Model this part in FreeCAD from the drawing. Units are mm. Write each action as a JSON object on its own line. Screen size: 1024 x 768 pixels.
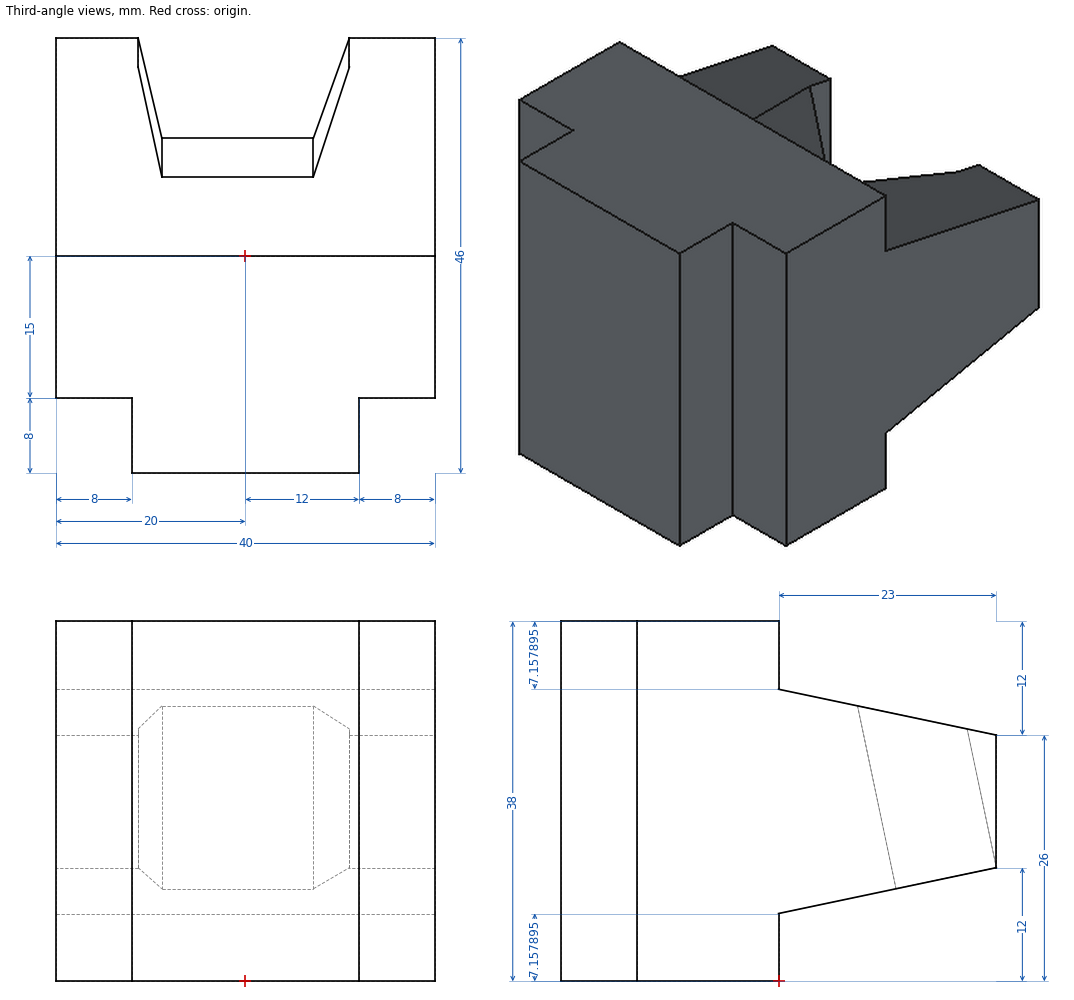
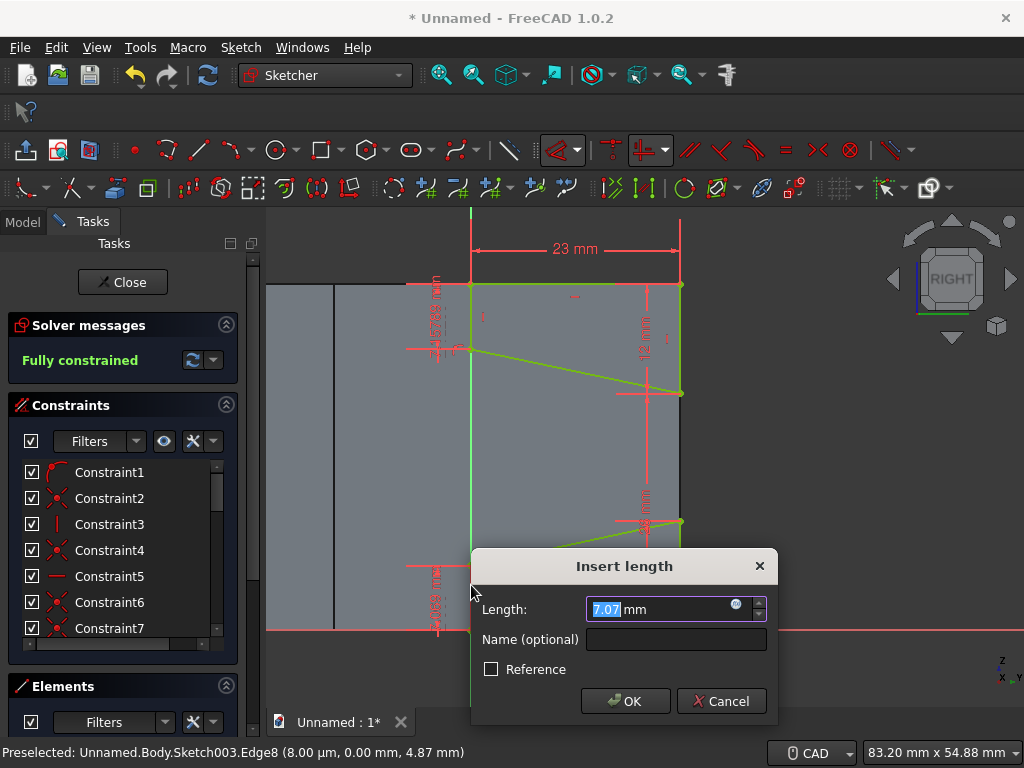
{"action": "type", "text": "7.157895"}
{"action": "key", "text": "Return"}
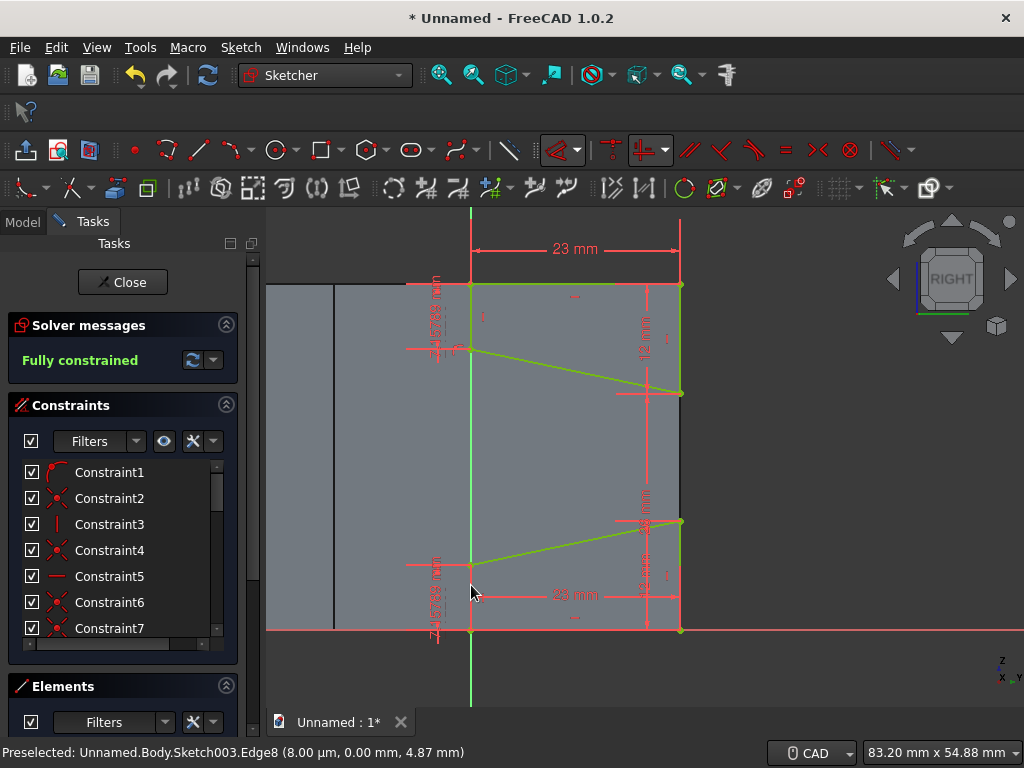
{"action": "left_click", "coordinate": [123, 282]}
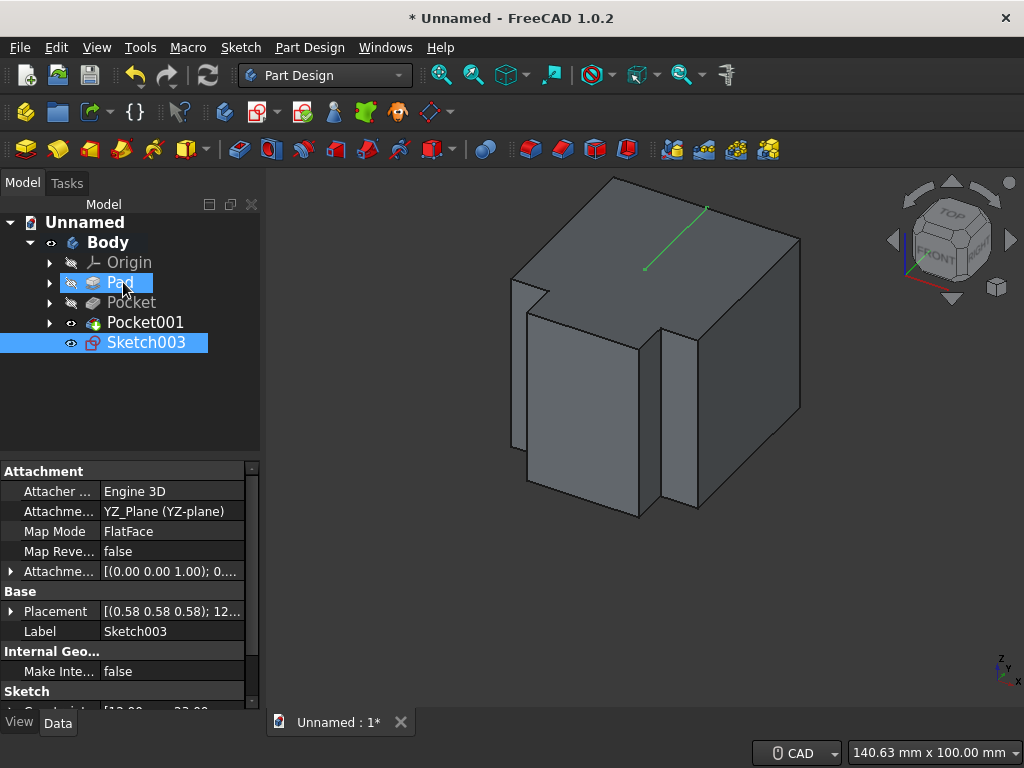
{"action": "left_click", "coordinate": [240, 150]}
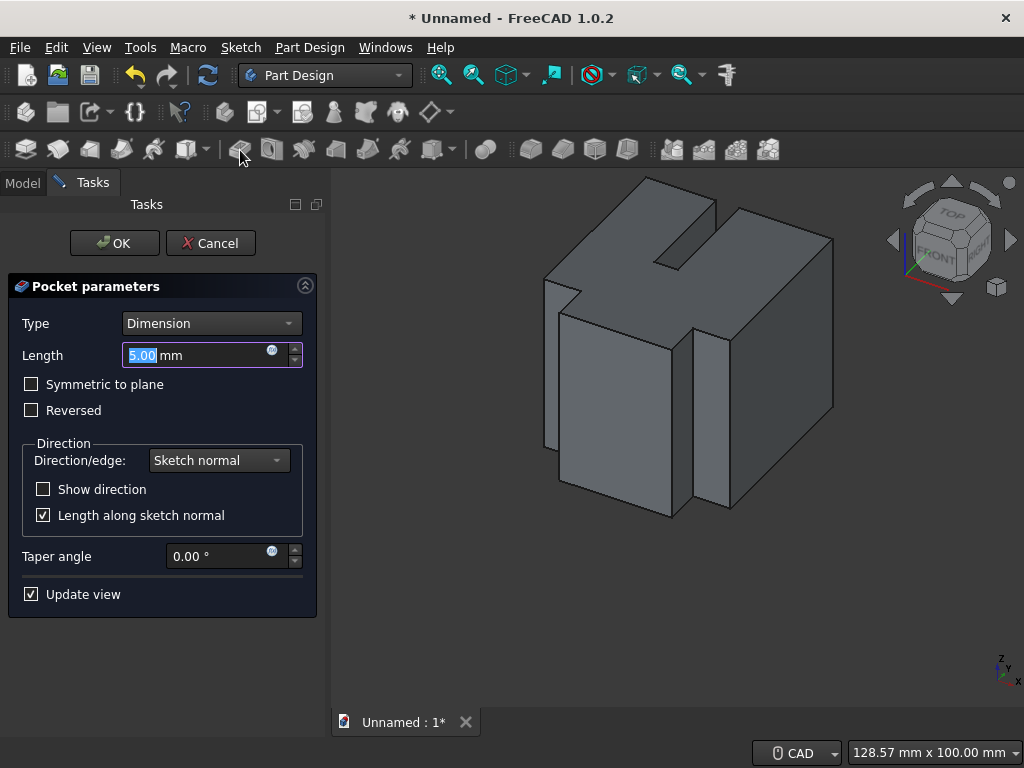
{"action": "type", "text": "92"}
{"action": "key", "text": "Tab"}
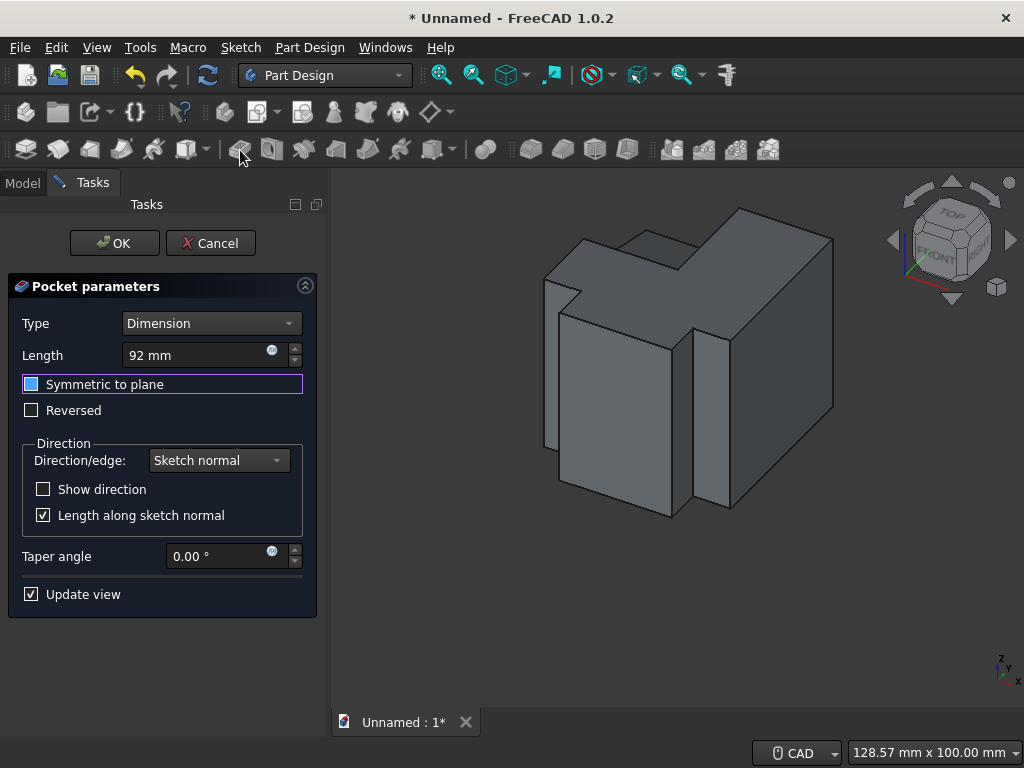
{"action": "left_click", "coordinate": [30, 384]}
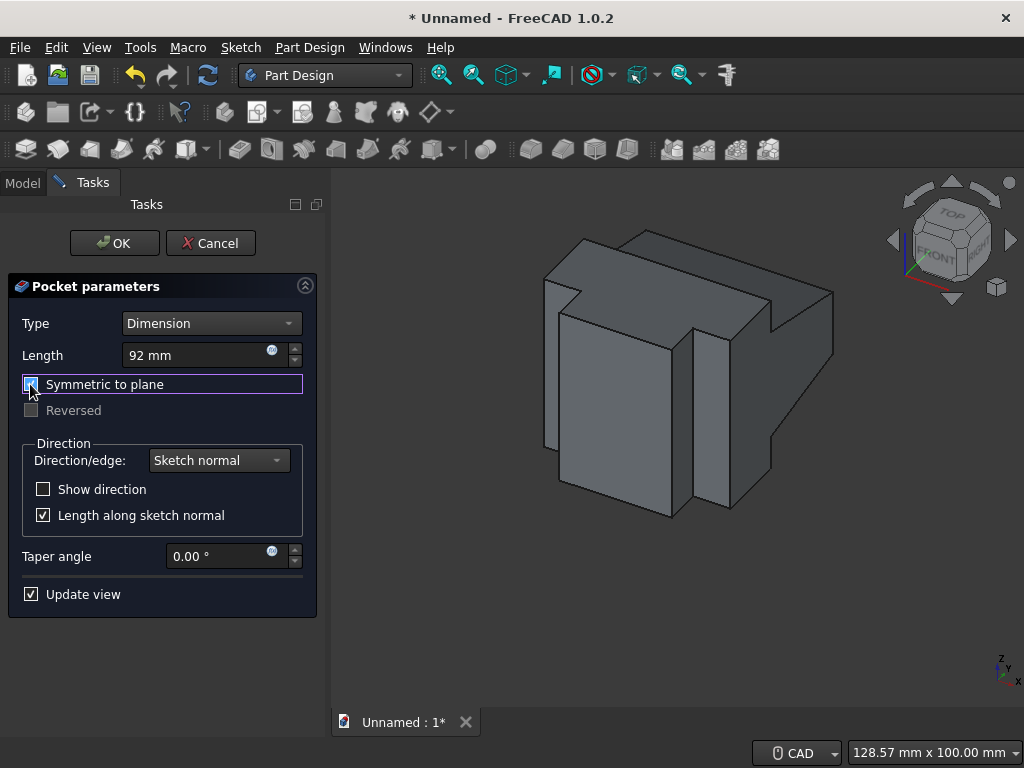
{"action": "left_click", "coordinate": [115, 243]}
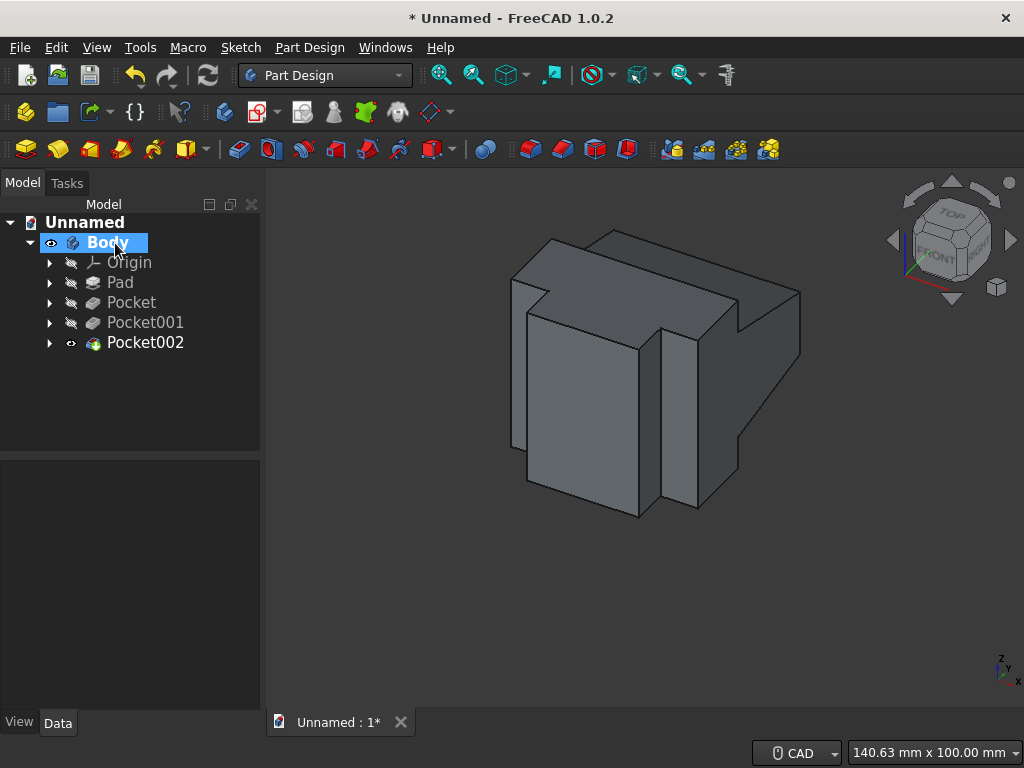
{"action": "key", "text": "5"}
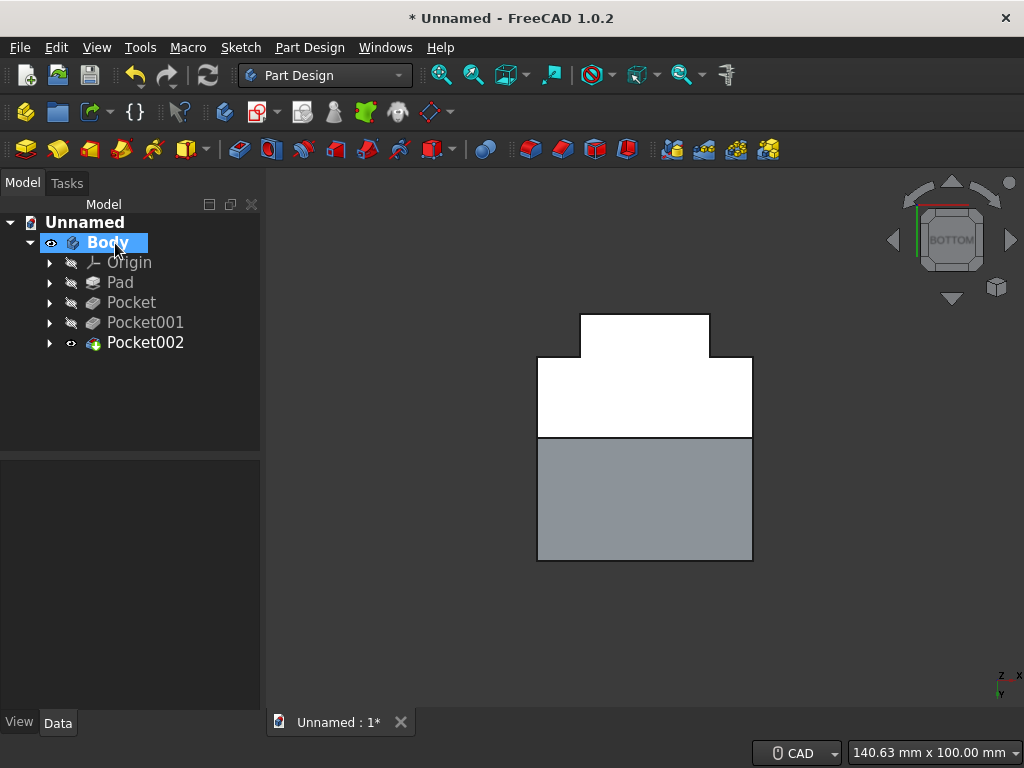
{"action": "left_click", "coordinate": [676, 498]}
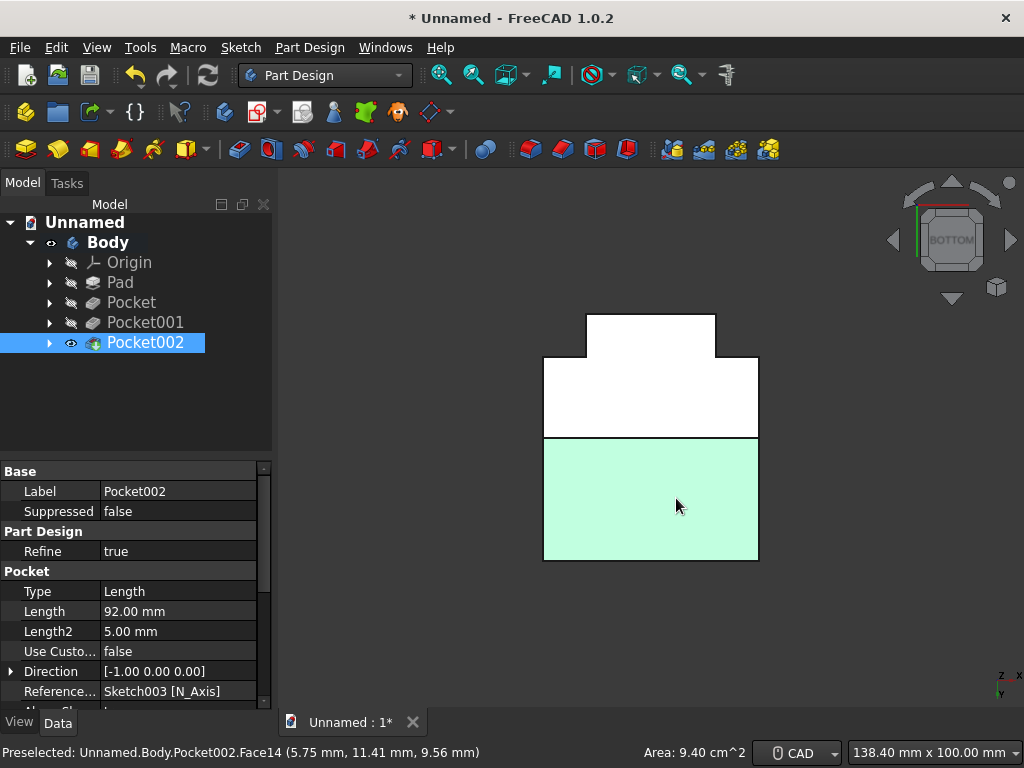
{"action": "left_click", "coordinate": [258, 112]}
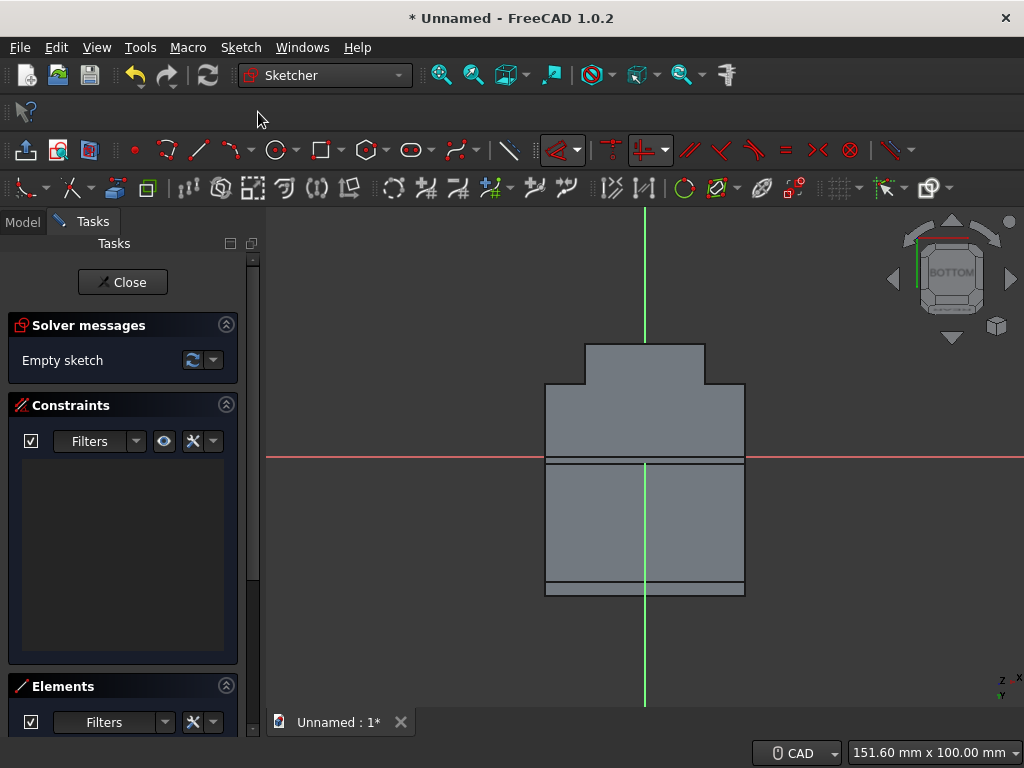
{"action": "scroll", "coordinate": [684, 556], "scroll_direction": "up", "scroll_amount": 5}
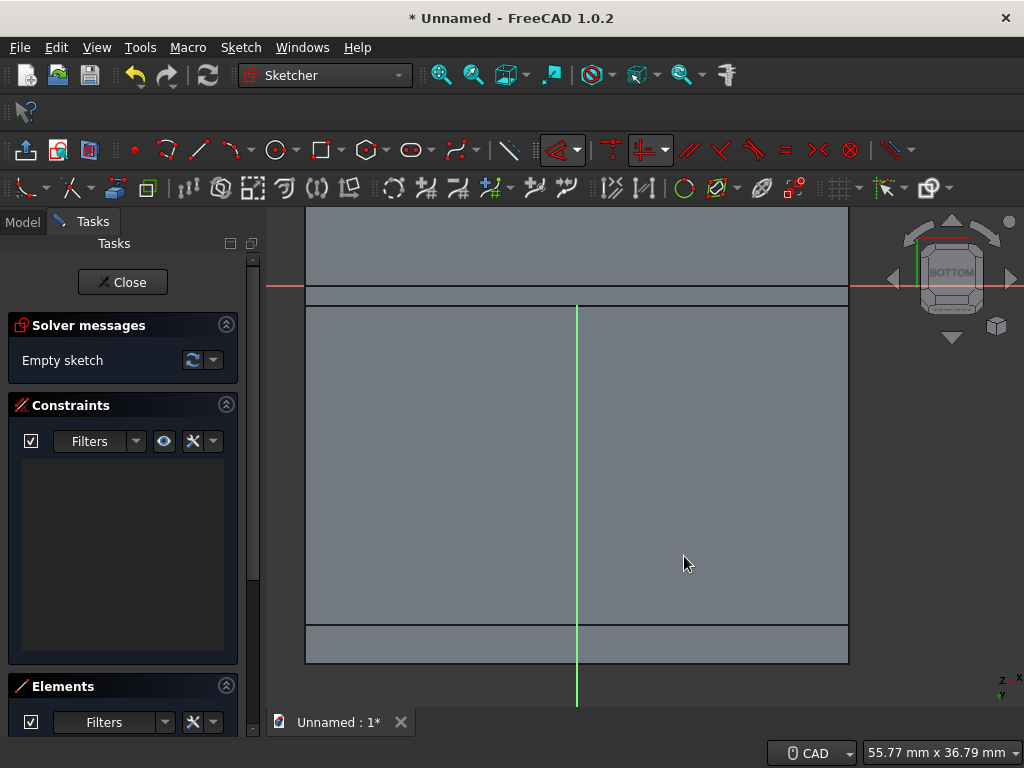
{"action": "left_click", "coordinate": [168, 150]}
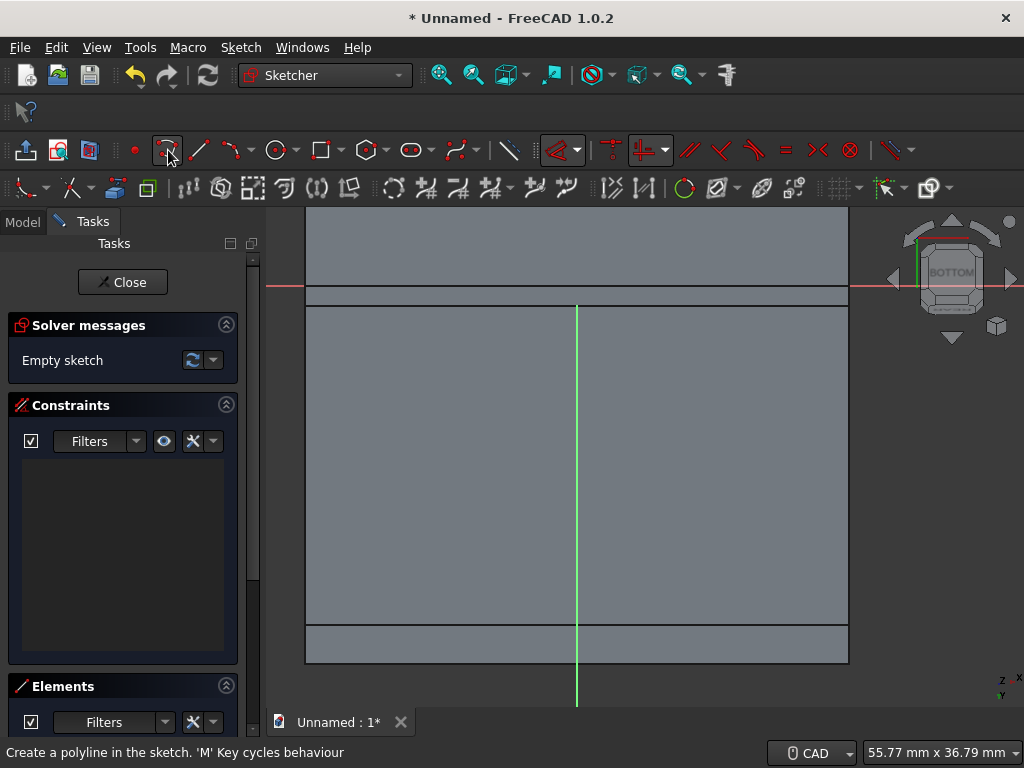
{"action": "left_click", "coordinate": [675, 478]}
{"action": "left_click", "coordinate": [457, 478]}
{"action": "left_click", "coordinate": [423, 625]}
{"action": "left_click", "coordinate": [726, 625]}
{"action": "left_click", "coordinate": [675, 479]}
{"action": "key", "text": "Escape"}
{"action": "key", "text": "Escape"}